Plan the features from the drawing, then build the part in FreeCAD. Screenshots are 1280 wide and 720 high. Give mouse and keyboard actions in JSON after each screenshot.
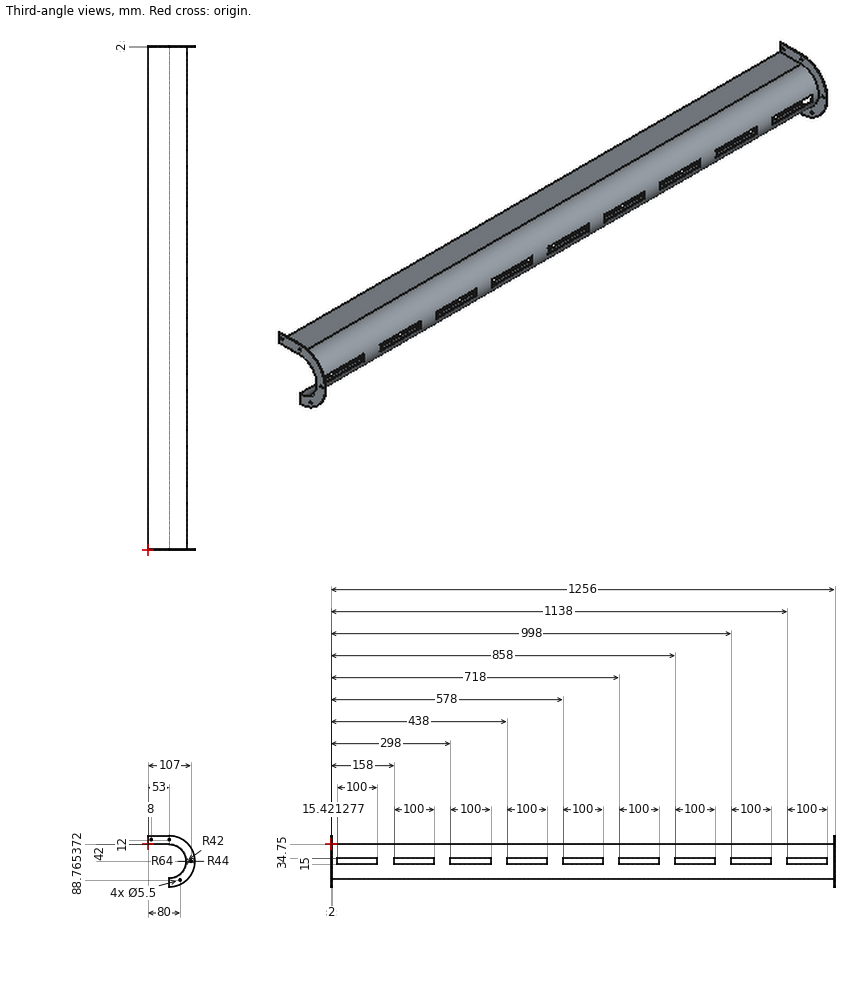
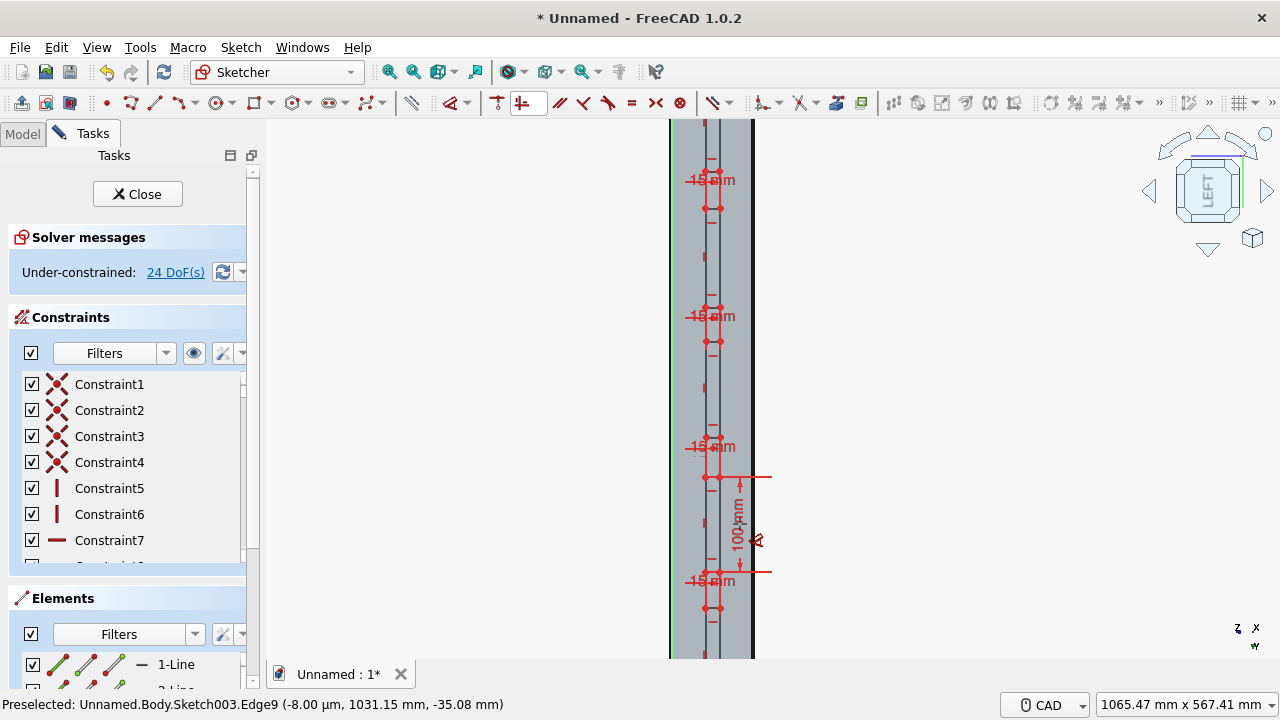
{"action": "scroll", "coordinate": [708, 508], "scroll_direction": "down", "scroll_amount": 6}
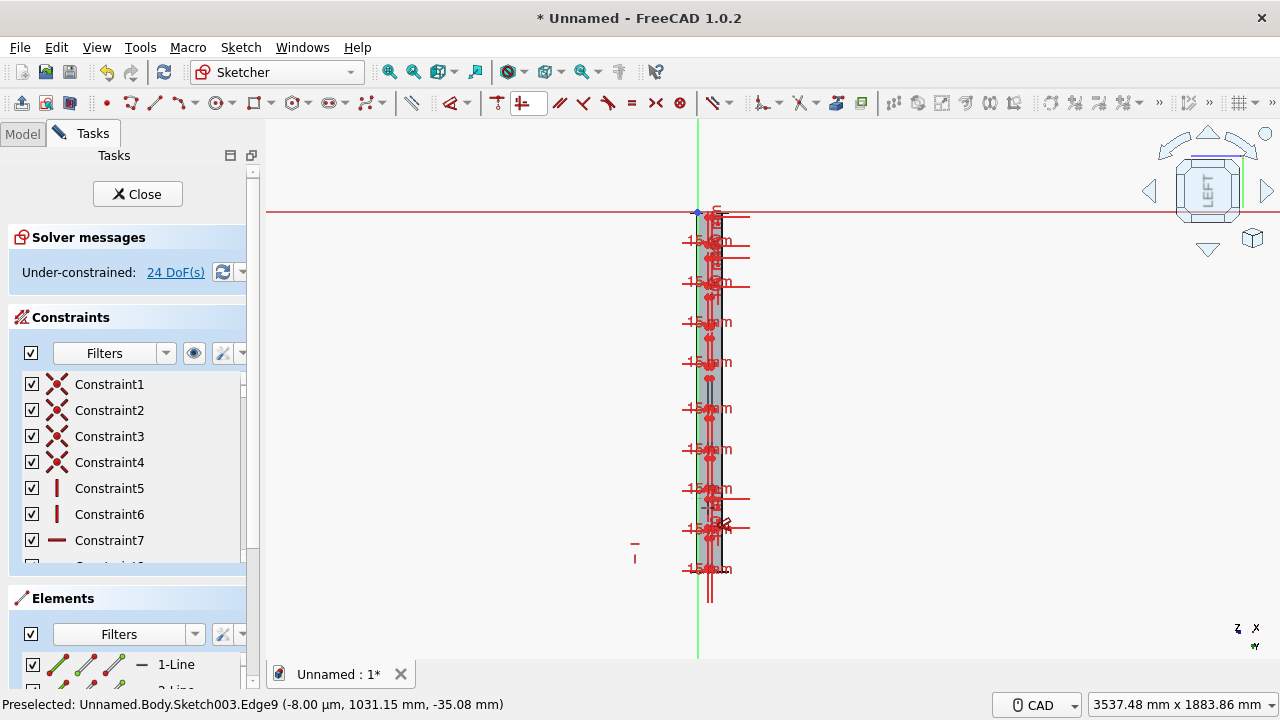
{"action": "scroll", "coordinate": [708, 307], "scroll_direction": "up", "scroll_amount": 6}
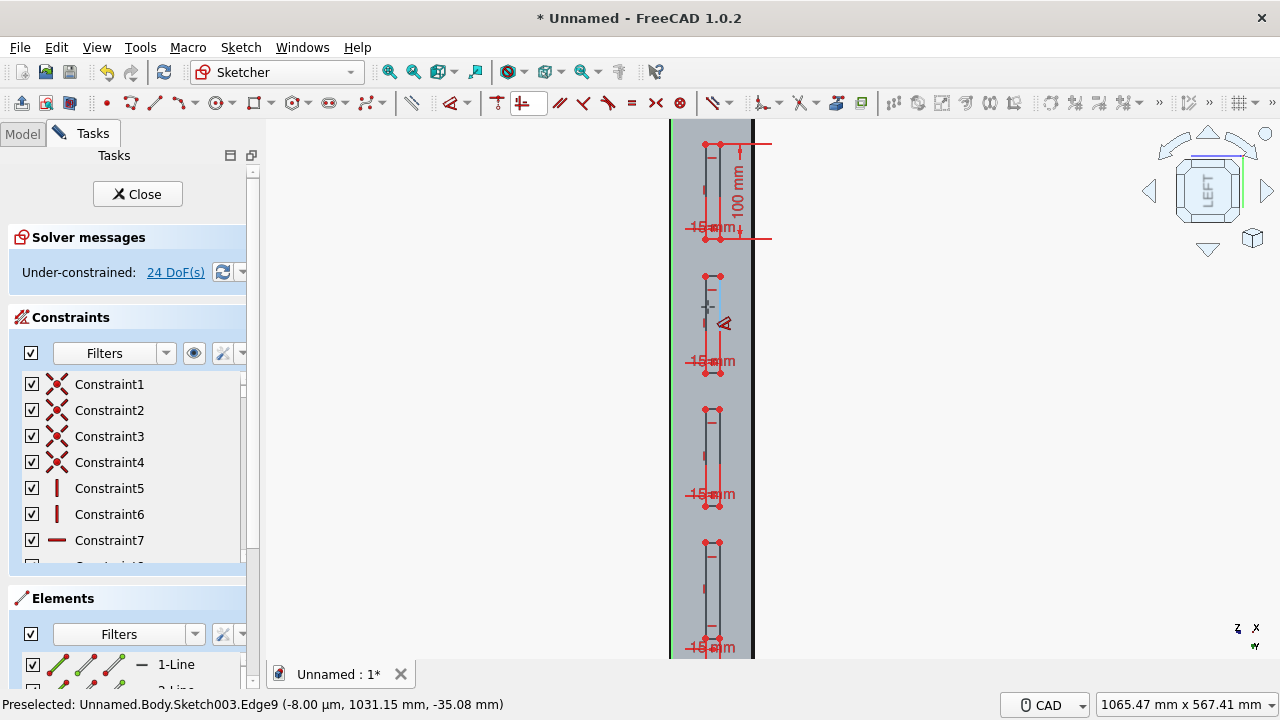
{"action": "left_click", "coordinate": [706, 305]}
{"action": "left_click", "coordinate": [740, 325]}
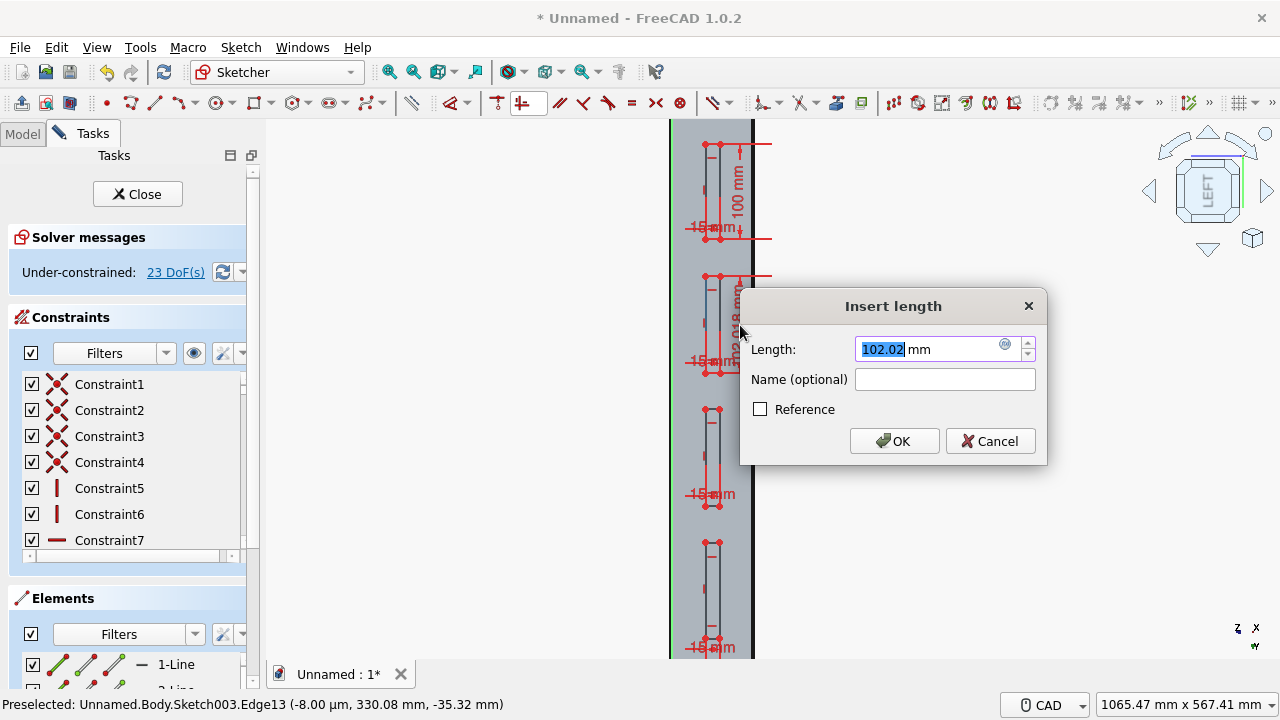
{"action": "type", "text": "100"}
{"action": "key", "text": "Return"}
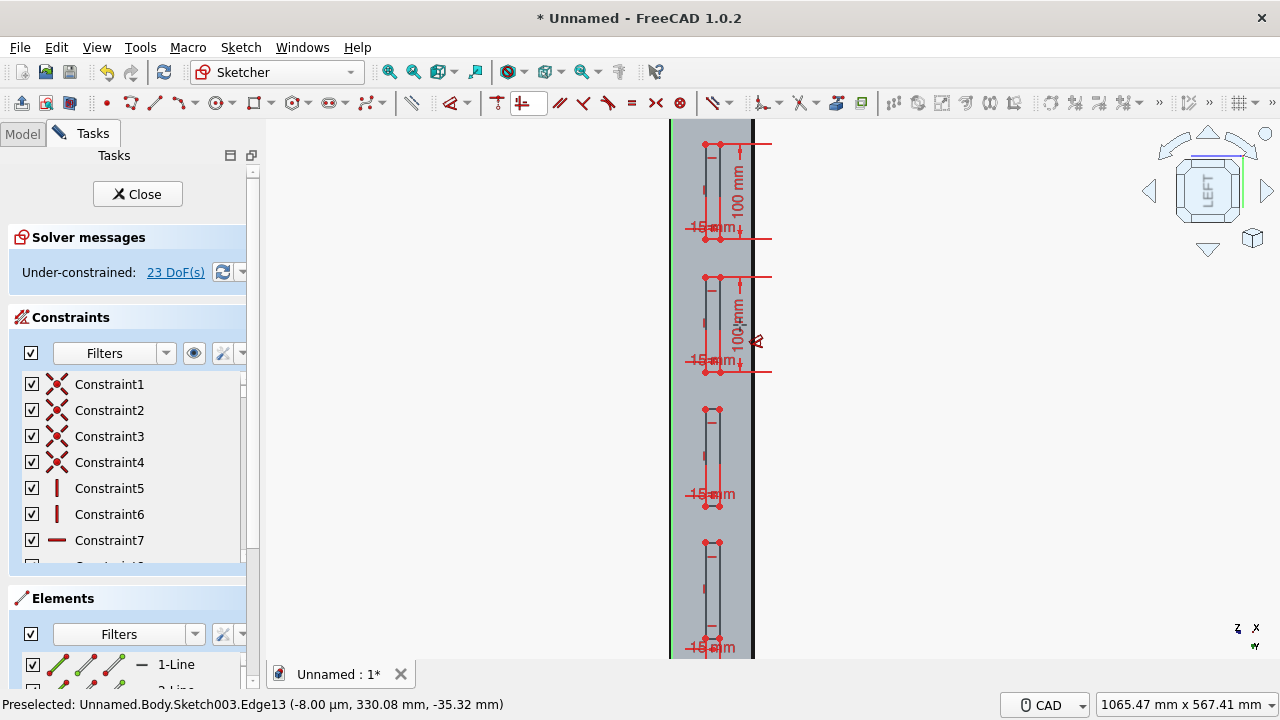
{"action": "left_click", "coordinate": [706, 438]}
{"action": "left_click", "coordinate": [740, 458]}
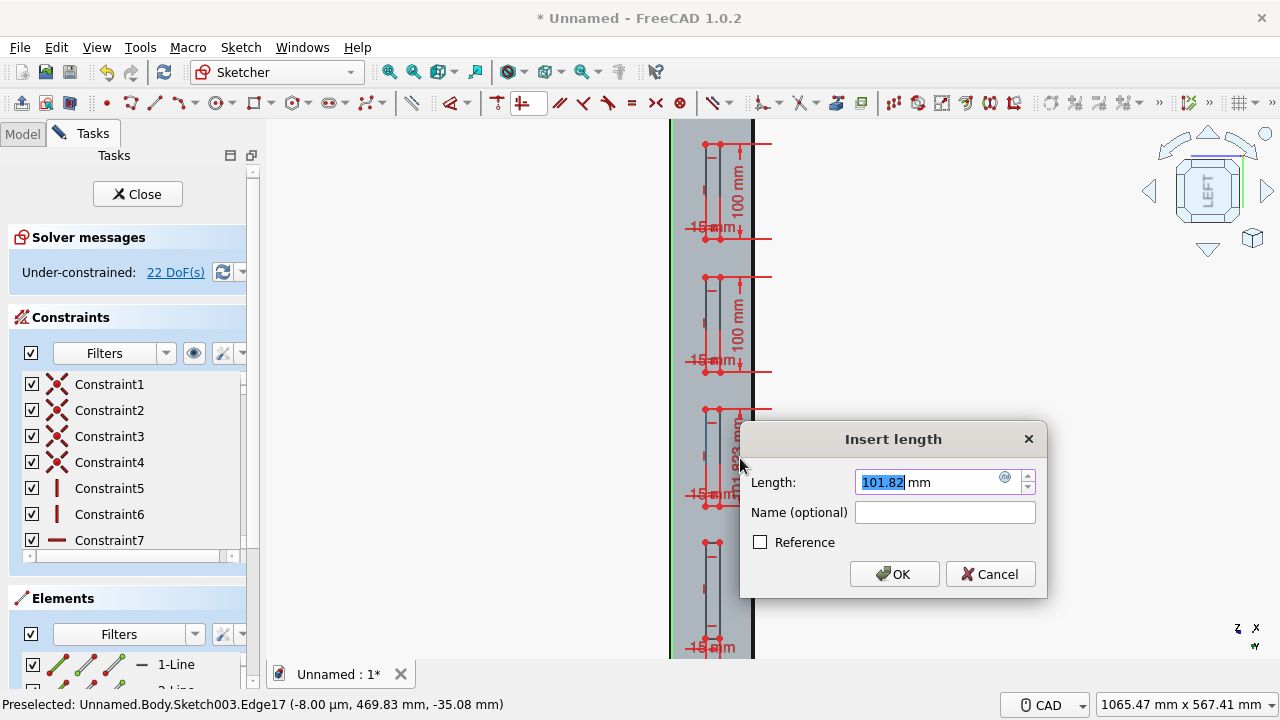
{"action": "type", "text": "100"}
{"action": "key", "text": "Return"}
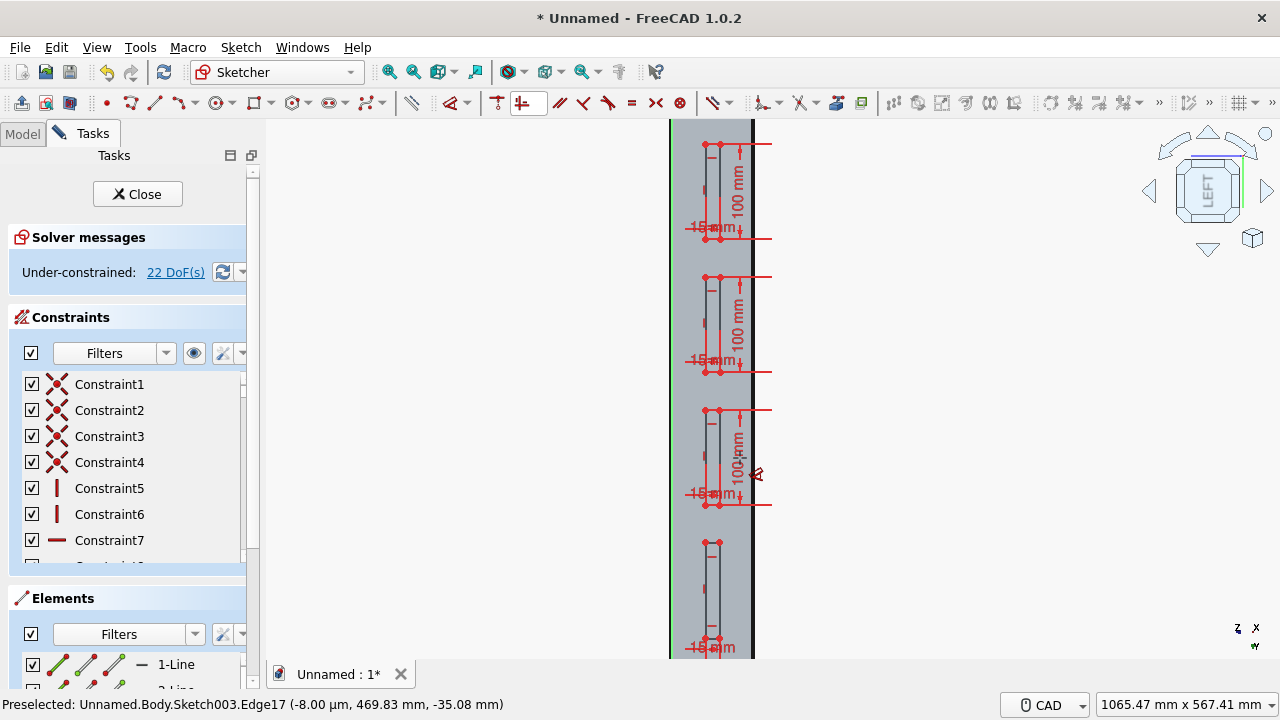
{"action": "left_click", "coordinate": [706, 572]}
{"action": "left_click", "coordinate": [740, 587]}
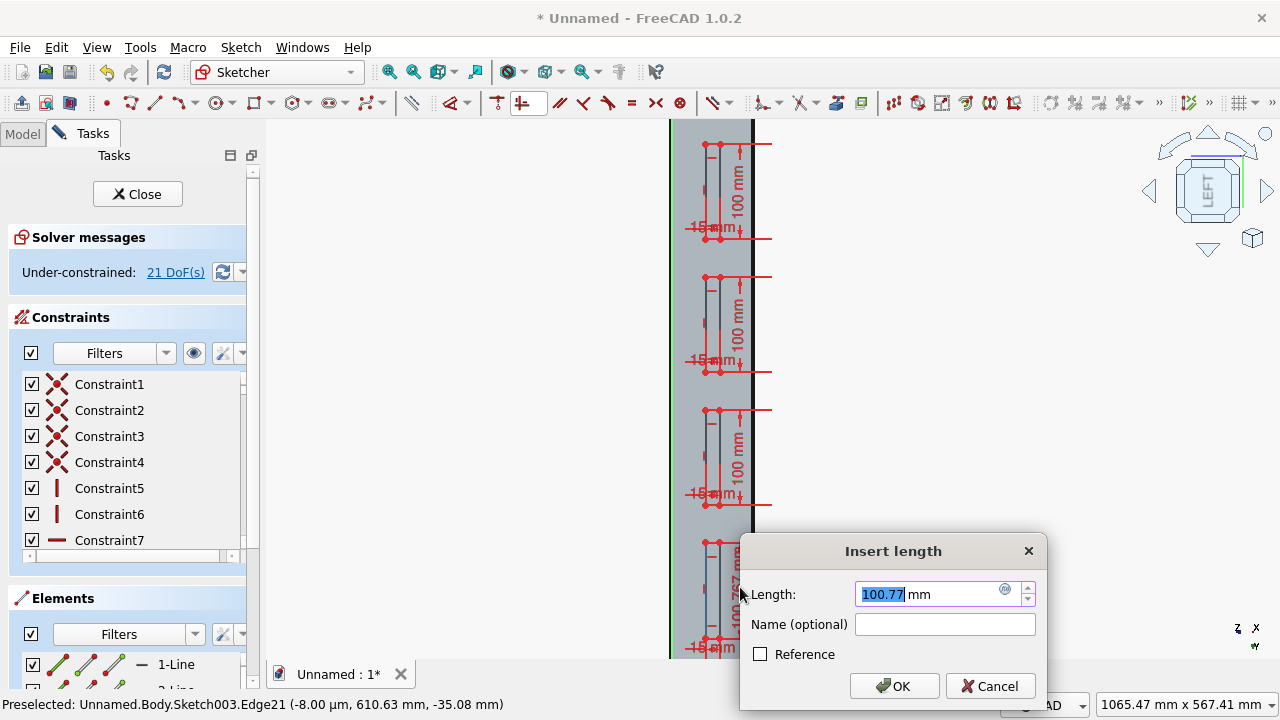
{"action": "type", "text": "100"}
{"action": "key", "text": "Return"}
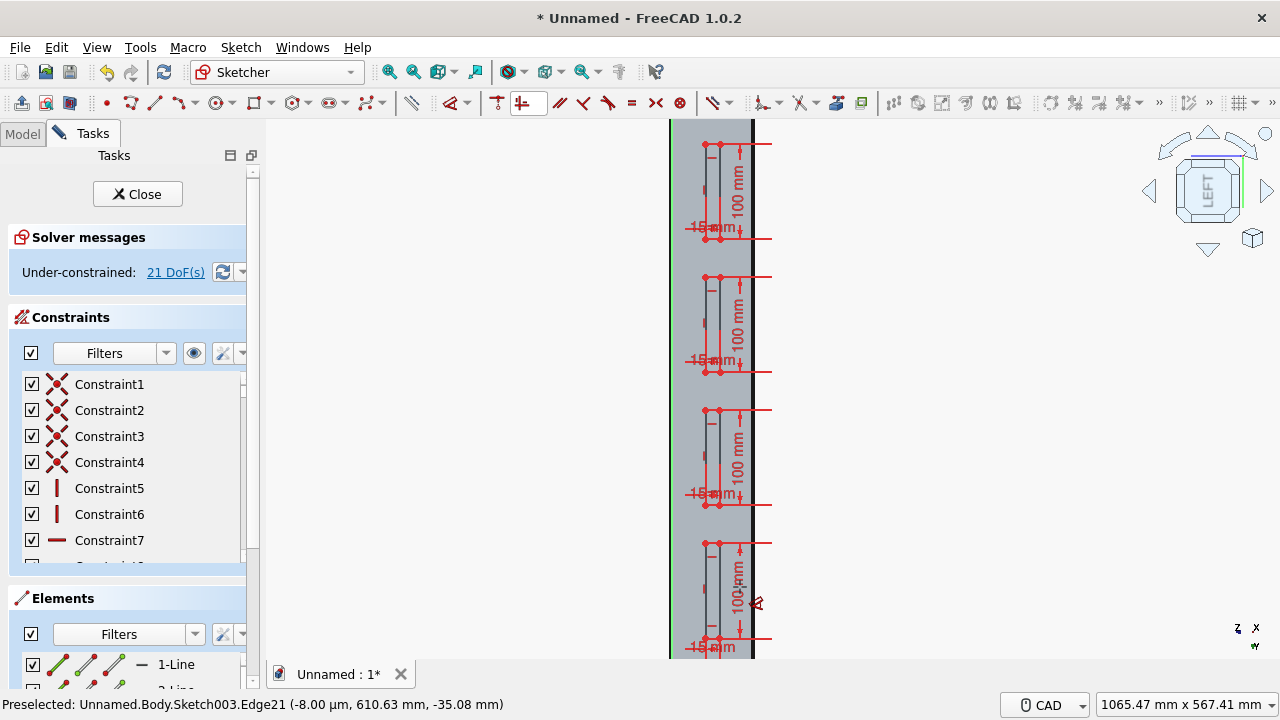
{"action": "scroll", "coordinate": [708, 306], "scroll_direction": "down", "scroll_amount": 6}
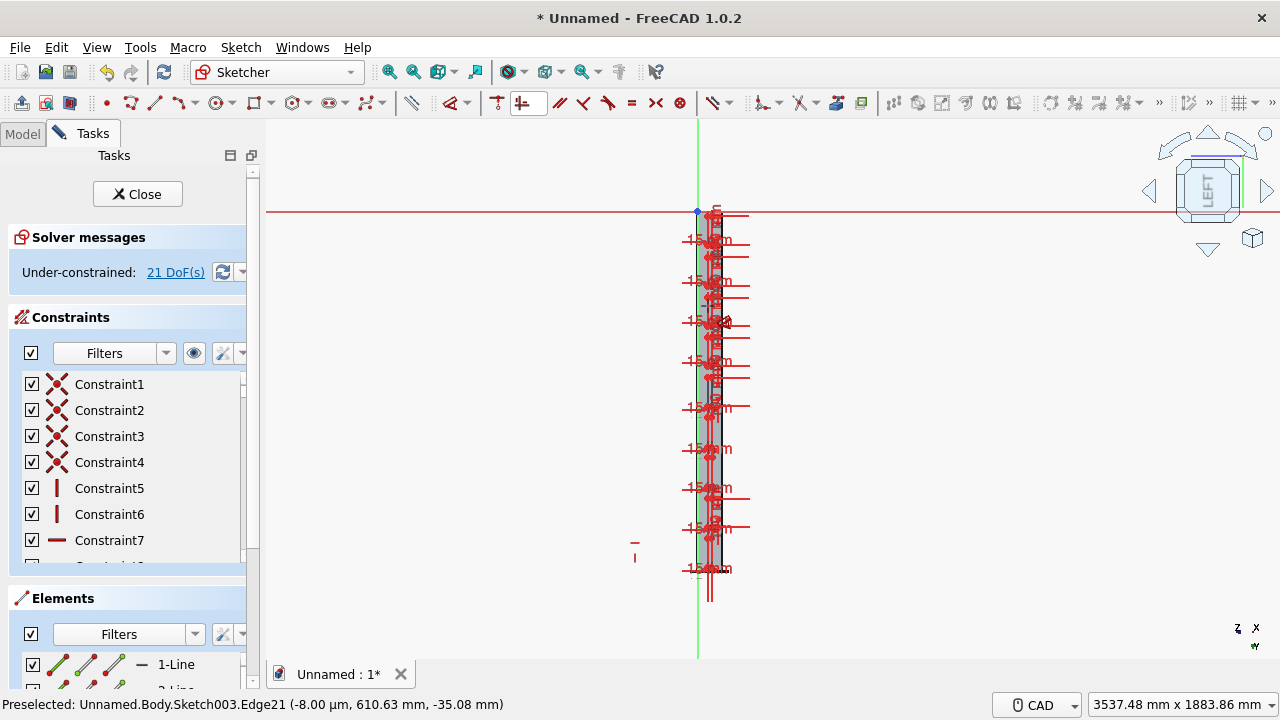
{"action": "scroll", "coordinate": [708, 427], "scroll_direction": "up", "scroll_amount": 6}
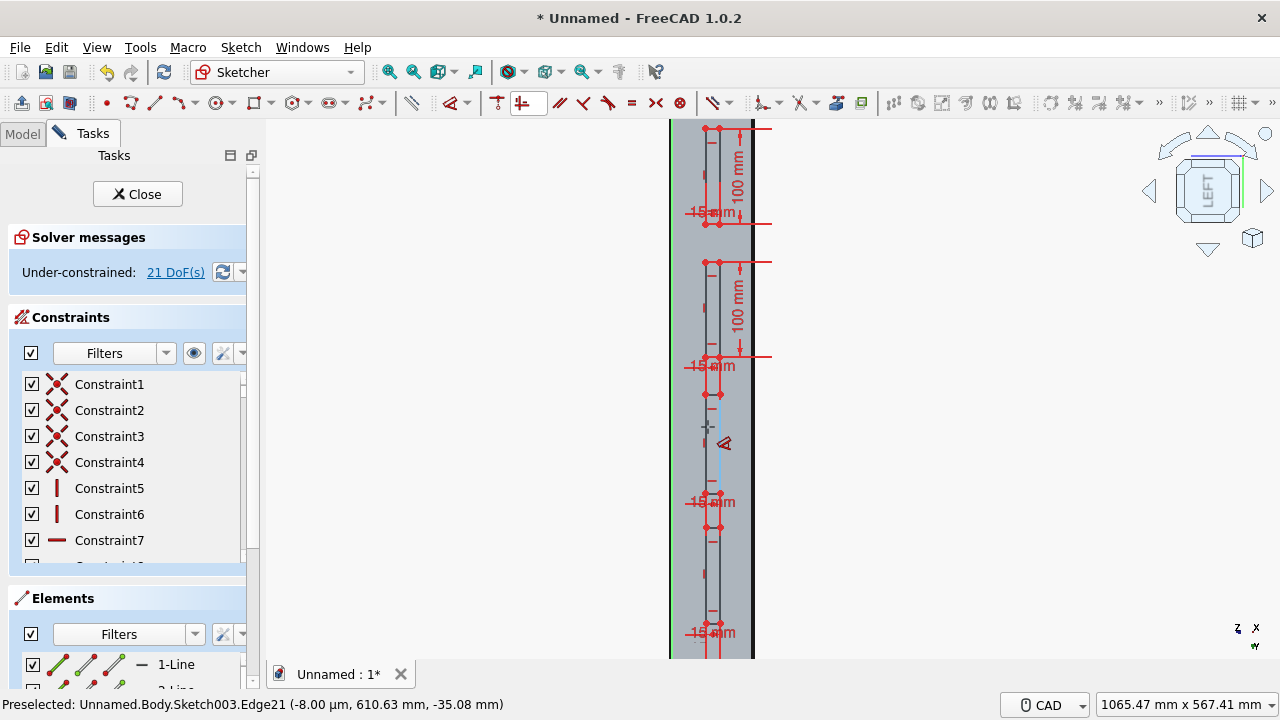
{"action": "left_click", "coordinate": [706, 424]}
{"action": "left_click", "coordinate": [740, 444]}